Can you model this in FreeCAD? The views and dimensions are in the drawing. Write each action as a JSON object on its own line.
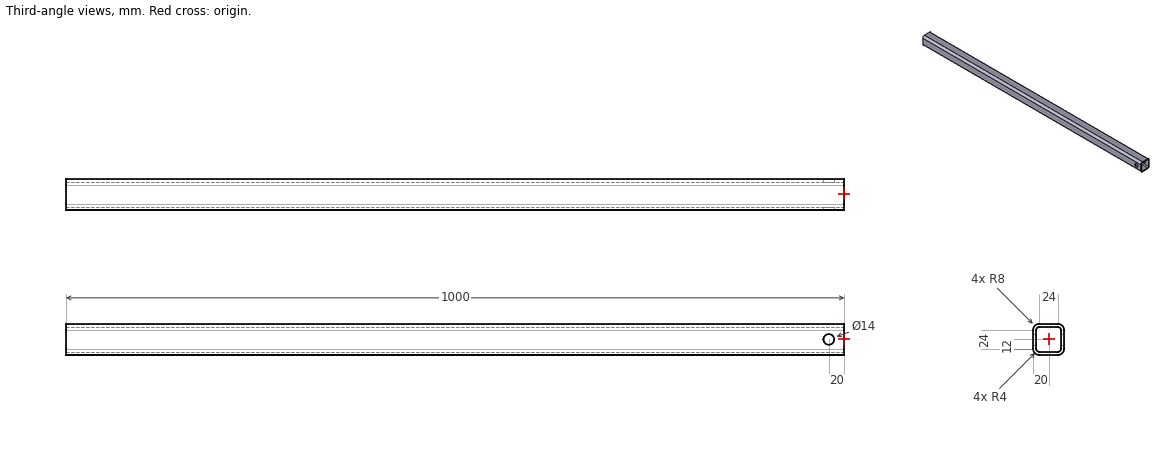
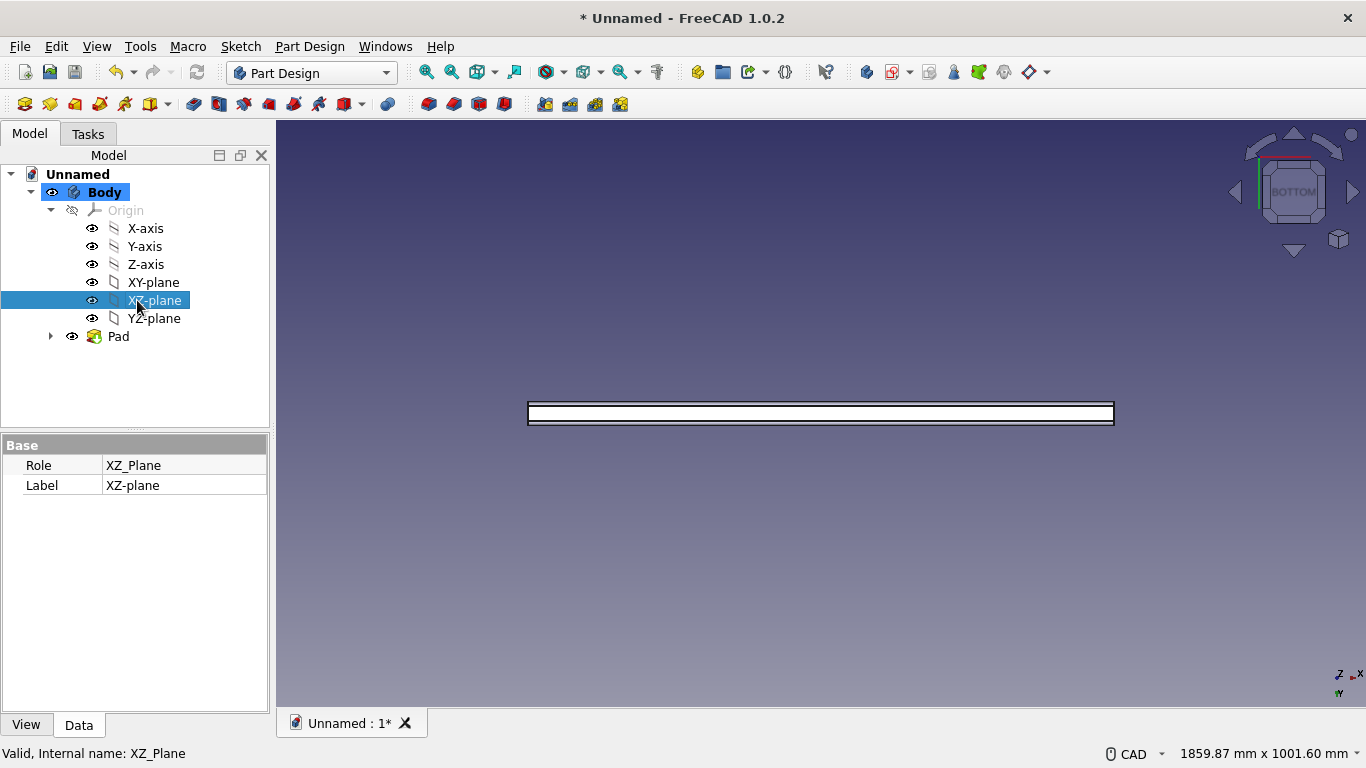
{"action": "left_click", "coordinate": [1028, 72]}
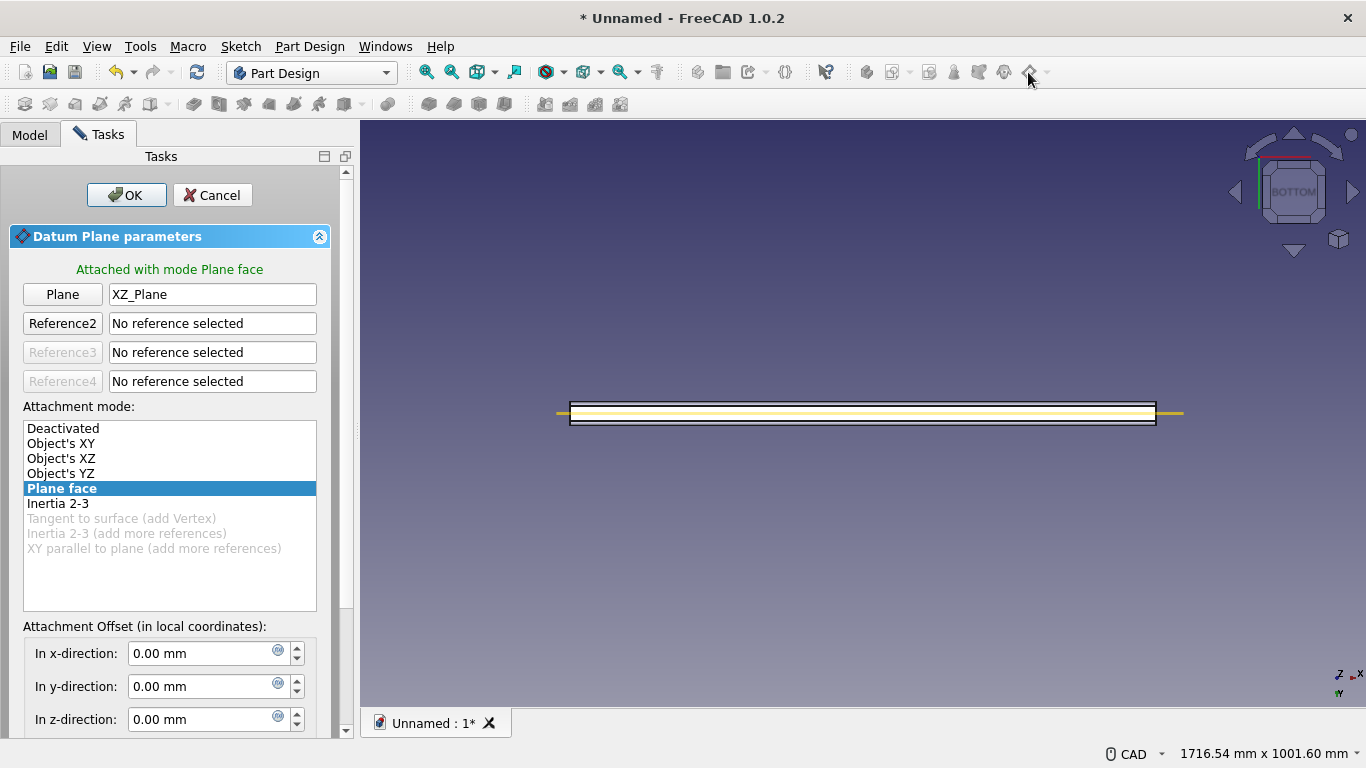
{"action": "triple_click", "coordinate": [210, 720]}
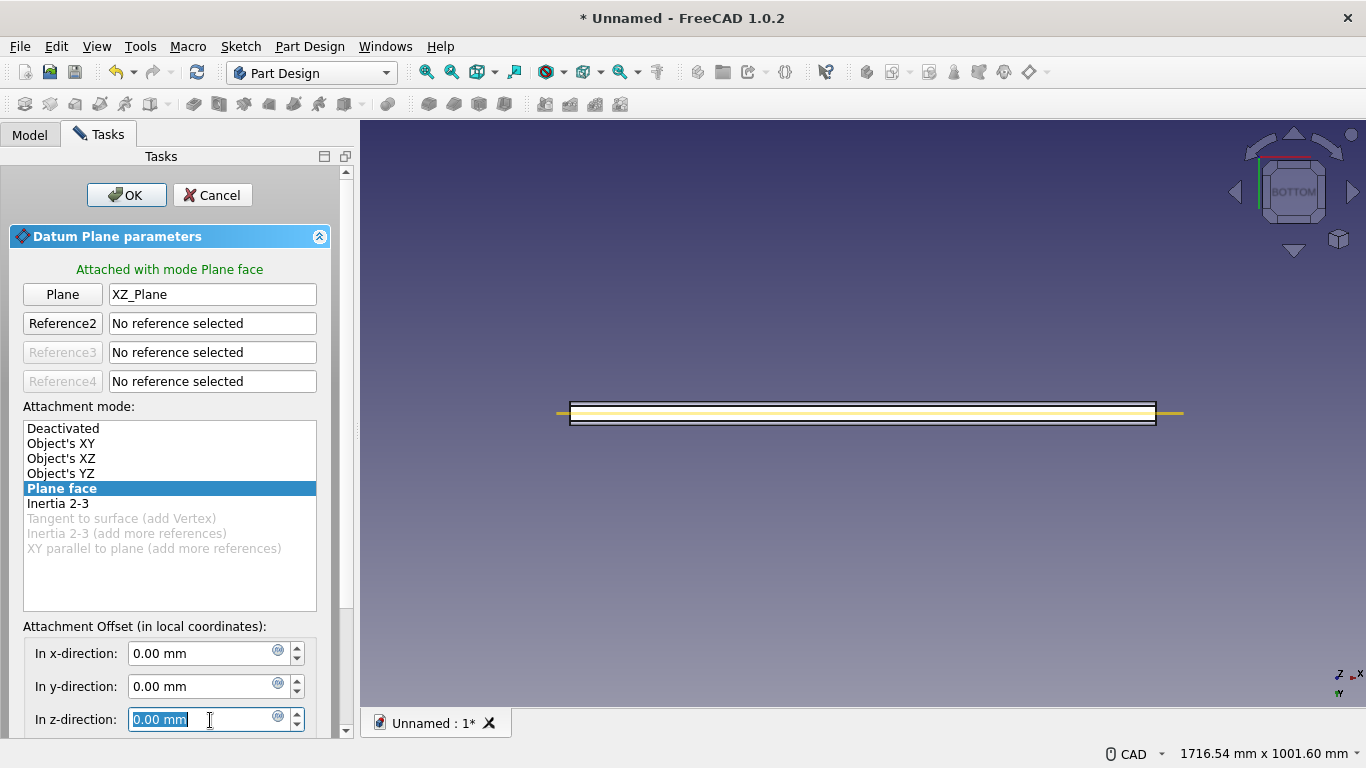
{"action": "type", "text": "-20"}
{"action": "key", "text": "Tab"}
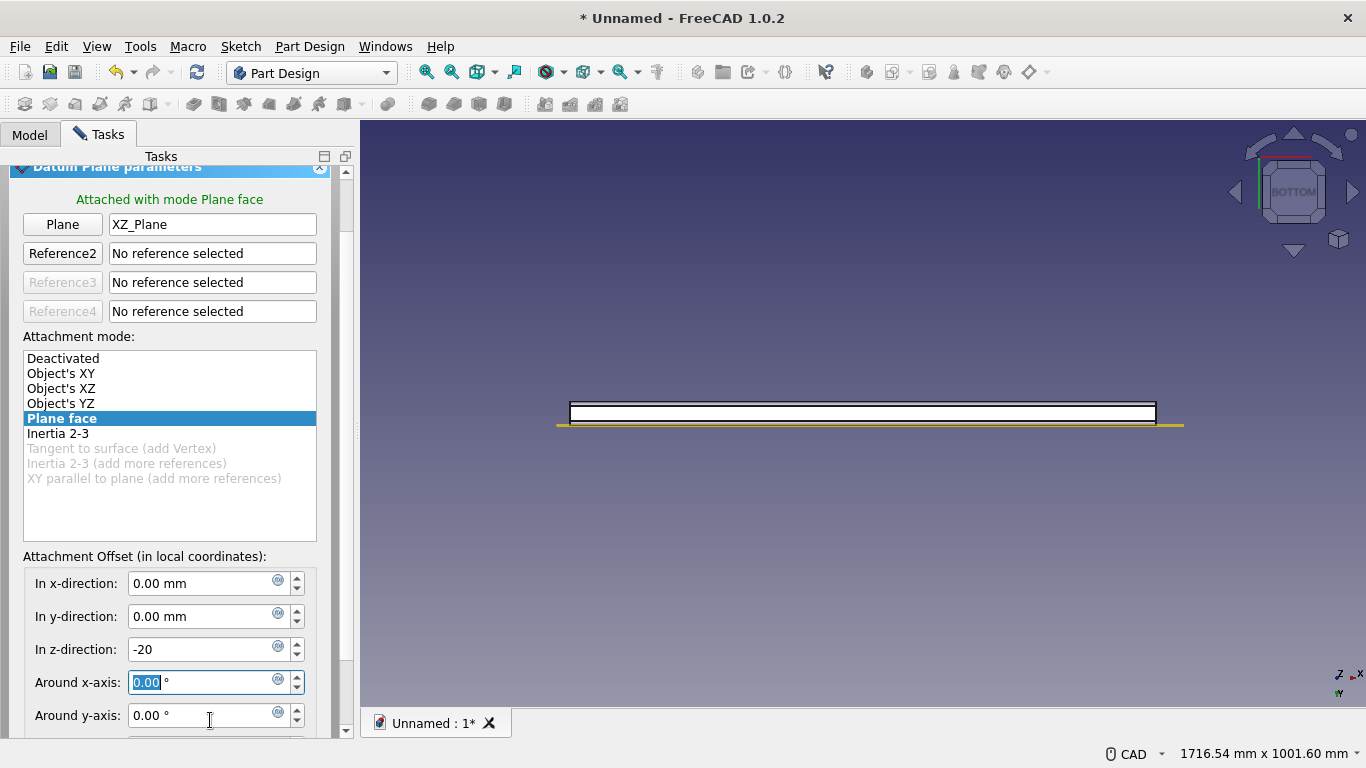
{"action": "scroll", "coordinate": [346, 452], "scroll_direction": "up", "scroll_amount": 2}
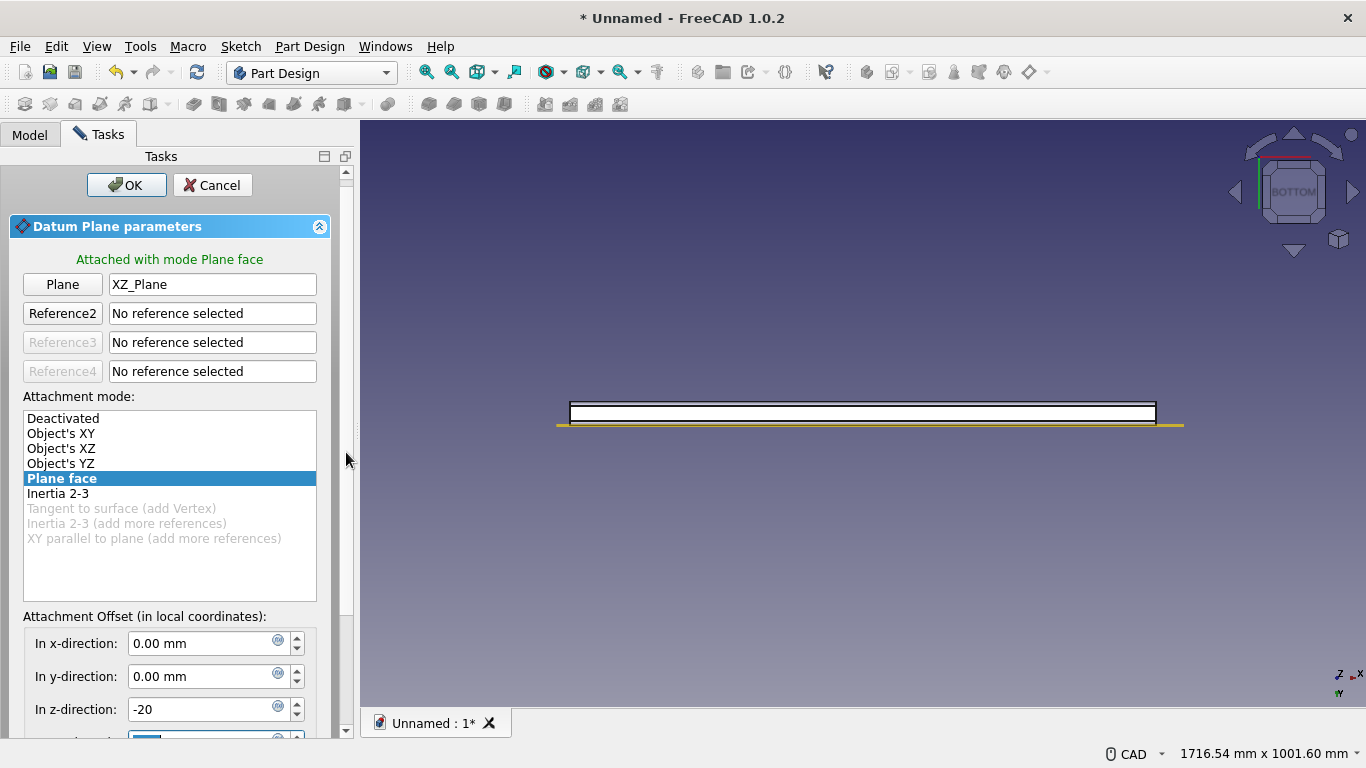
{"action": "left_click", "coordinate": [127, 195]}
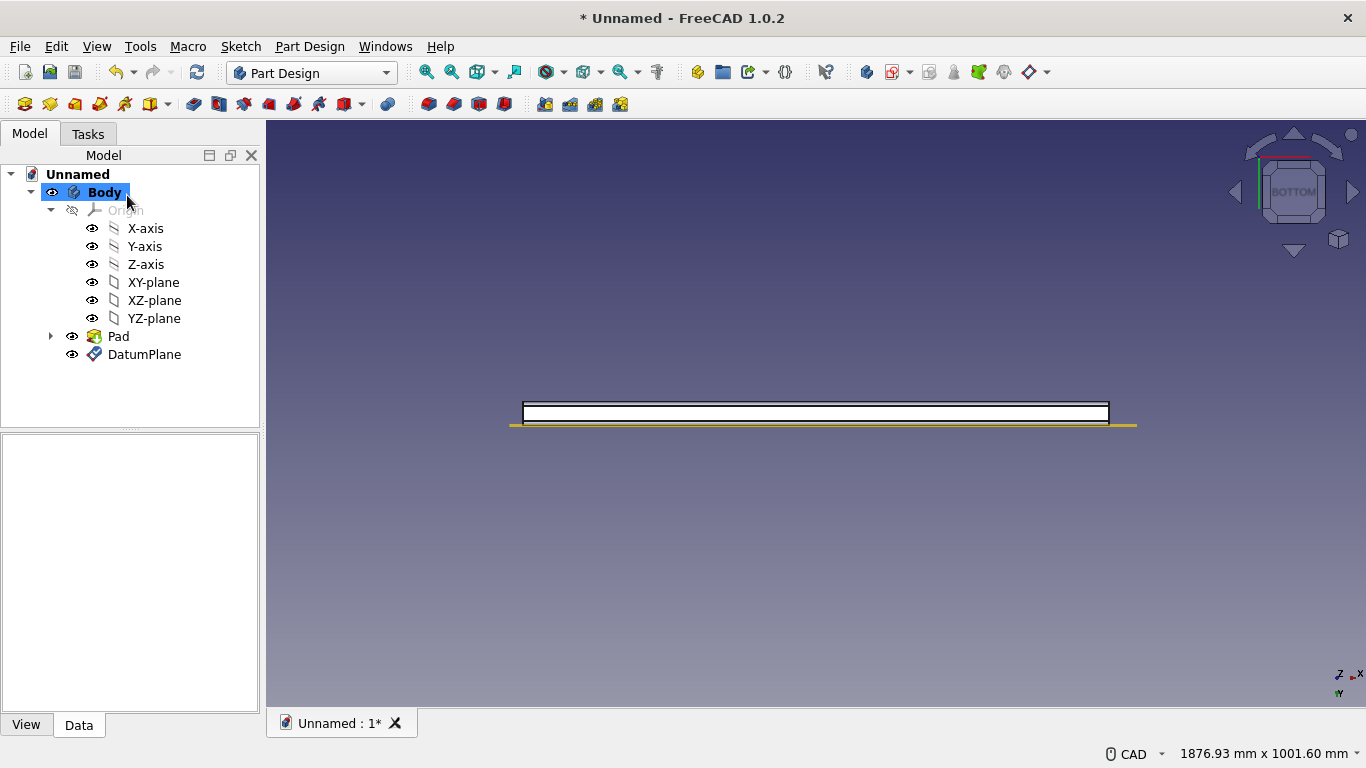
{"action": "left_click", "coordinate": [117, 354]}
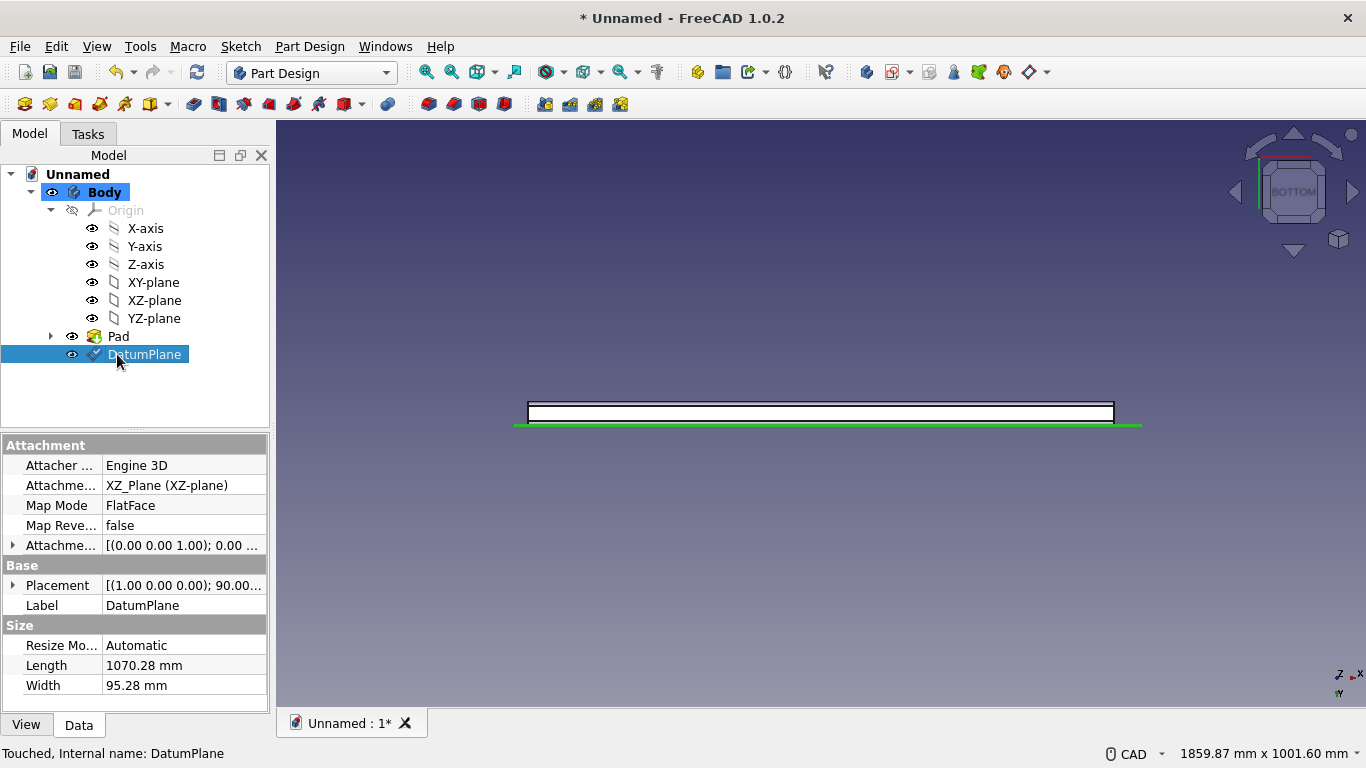
{"action": "left_click", "coordinate": [892, 72]}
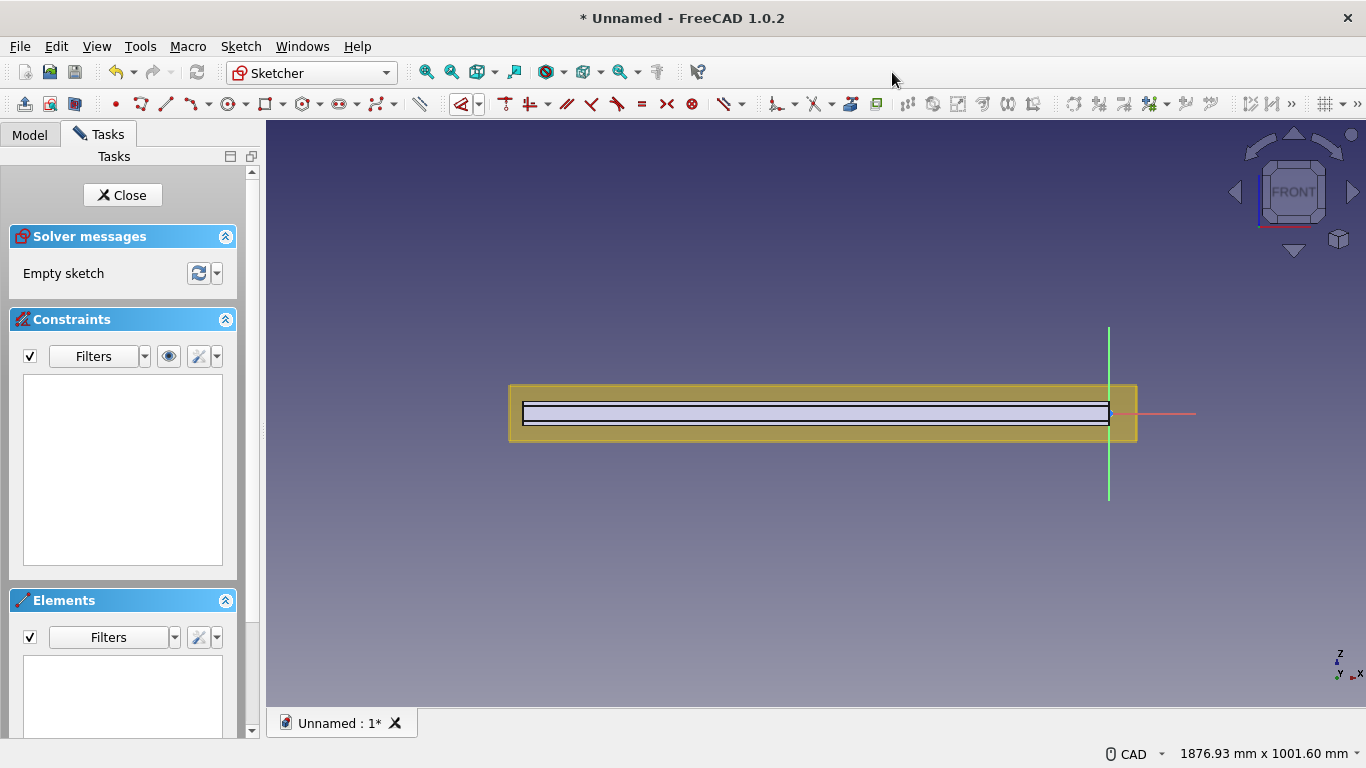
{"action": "left_click", "coordinate": [75, 104]}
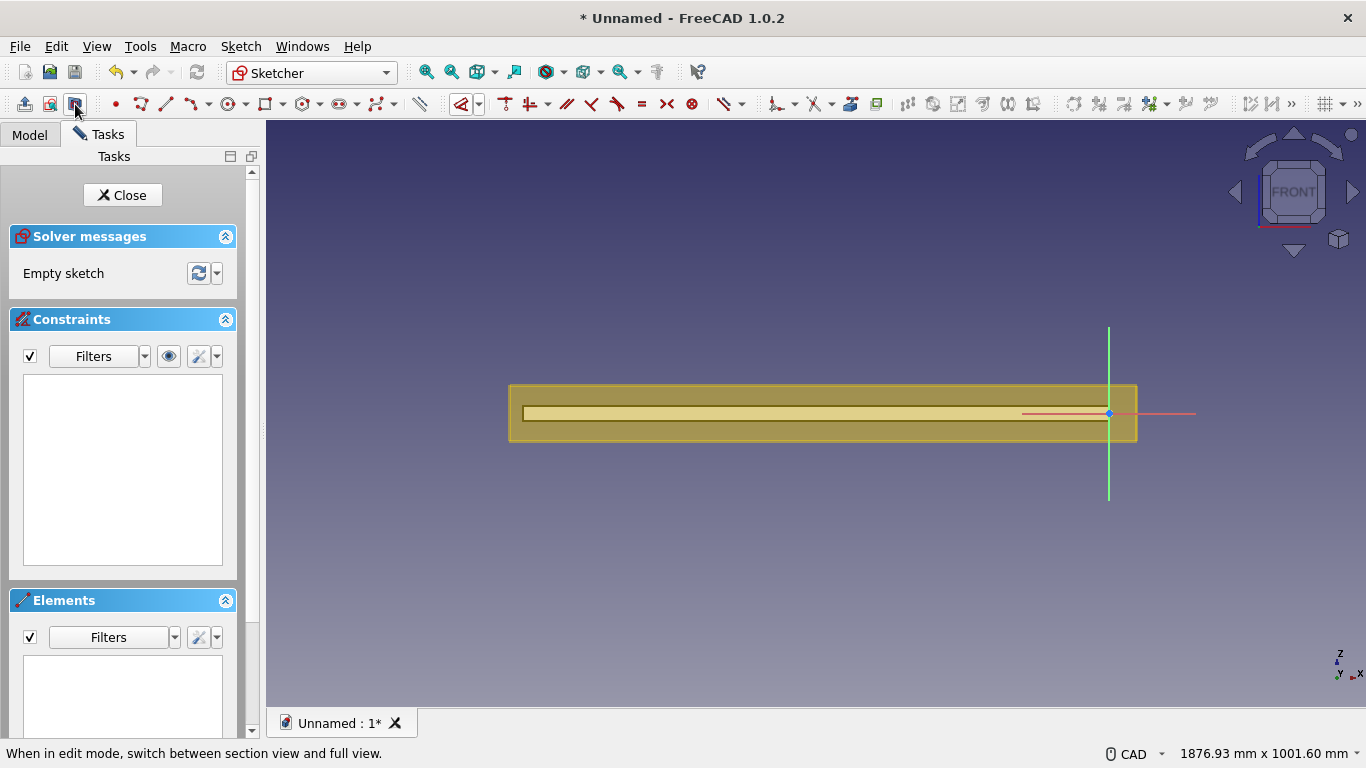
{"action": "scroll", "coordinate": [1120, 414], "scroll_direction": "up", "scroll_amount": 15}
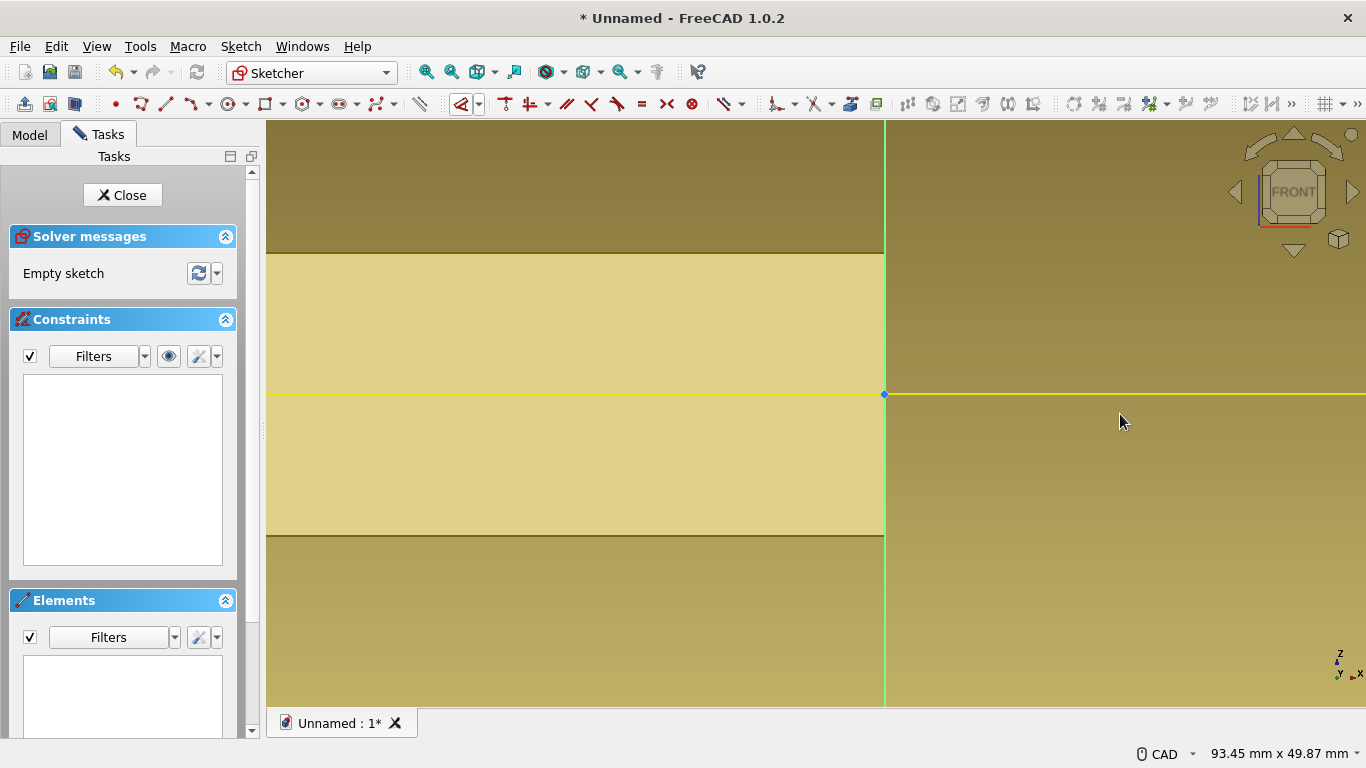
{"action": "scroll", "coordinate": [708, 379], "scroll_direction": "up", "scroll_amount": 4}